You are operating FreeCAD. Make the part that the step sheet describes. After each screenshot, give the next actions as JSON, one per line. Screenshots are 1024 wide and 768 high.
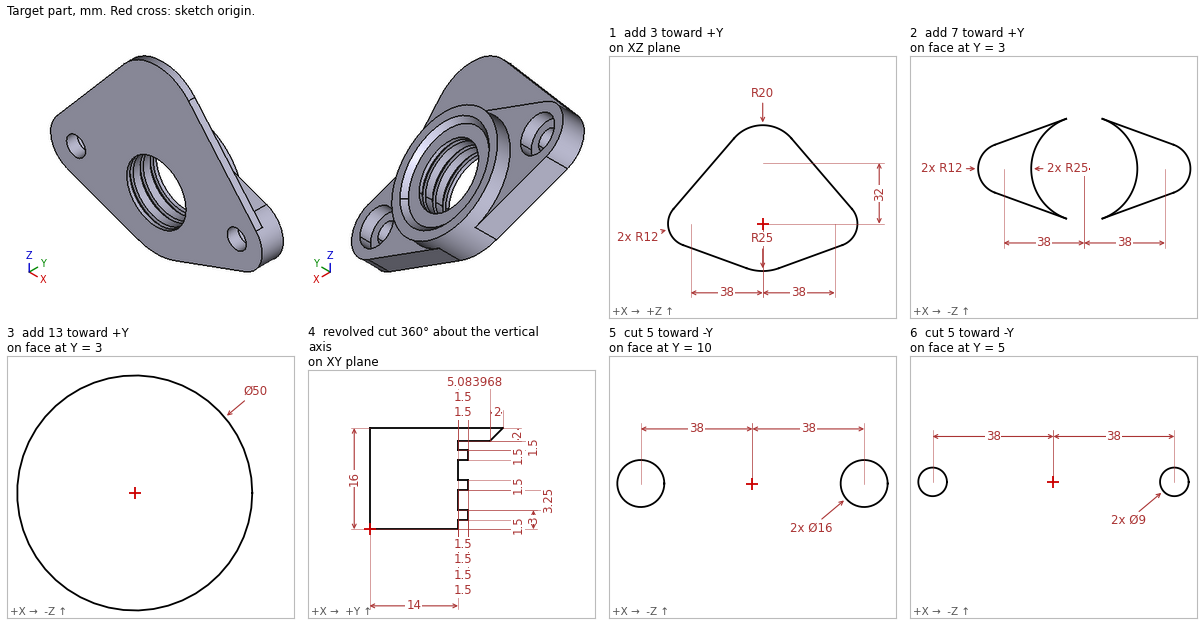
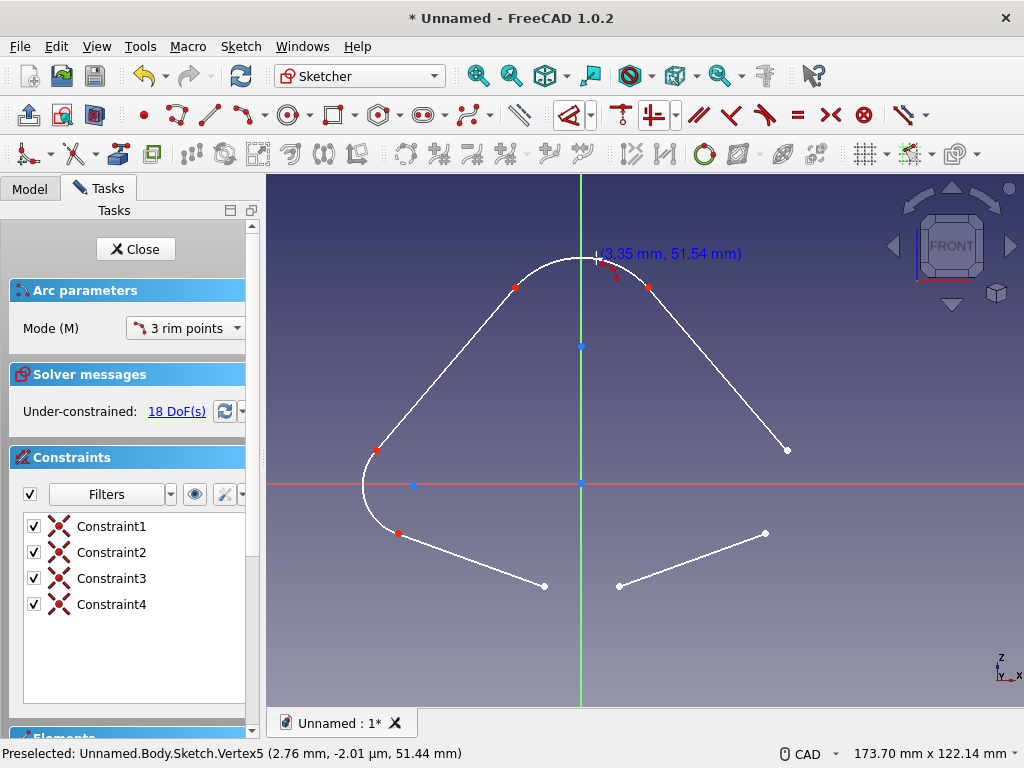
{"action": "left_click", "coordinate": [787, 451]}
{"action": "left_click", "coordinate": [765, 534]}
{"action": "left_click", "coordinate": [794, 507]}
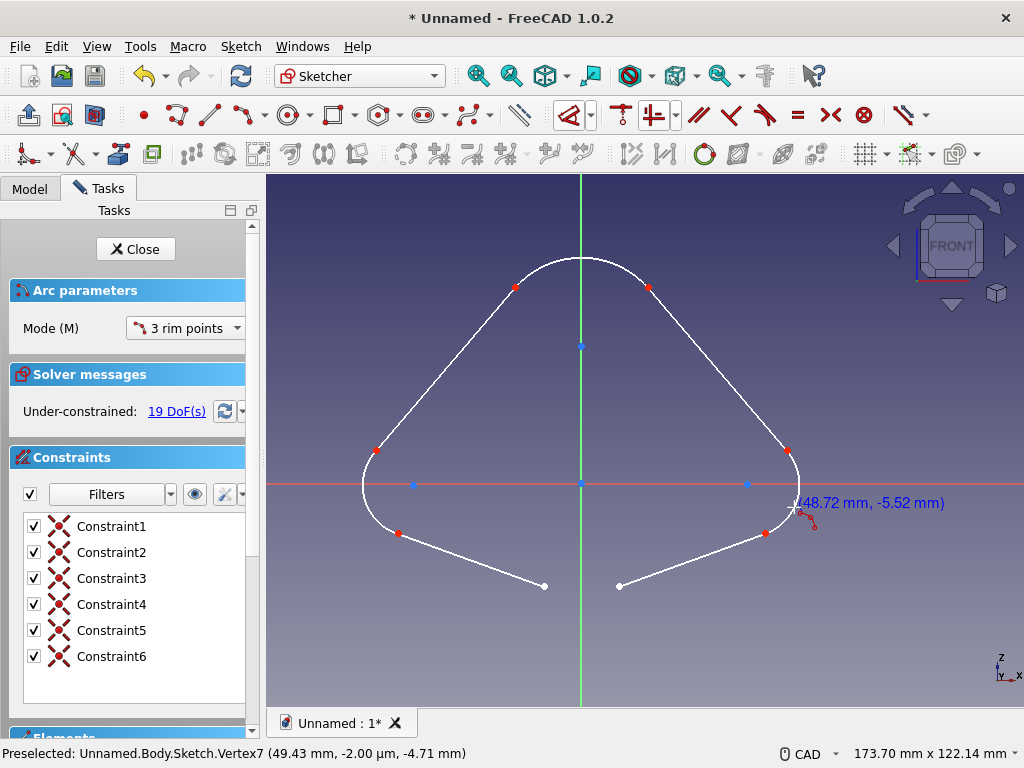
{"action": "left_click", "coordinate": [619, 587]}
{"action": "left_click", "coordinate": [544, 587]}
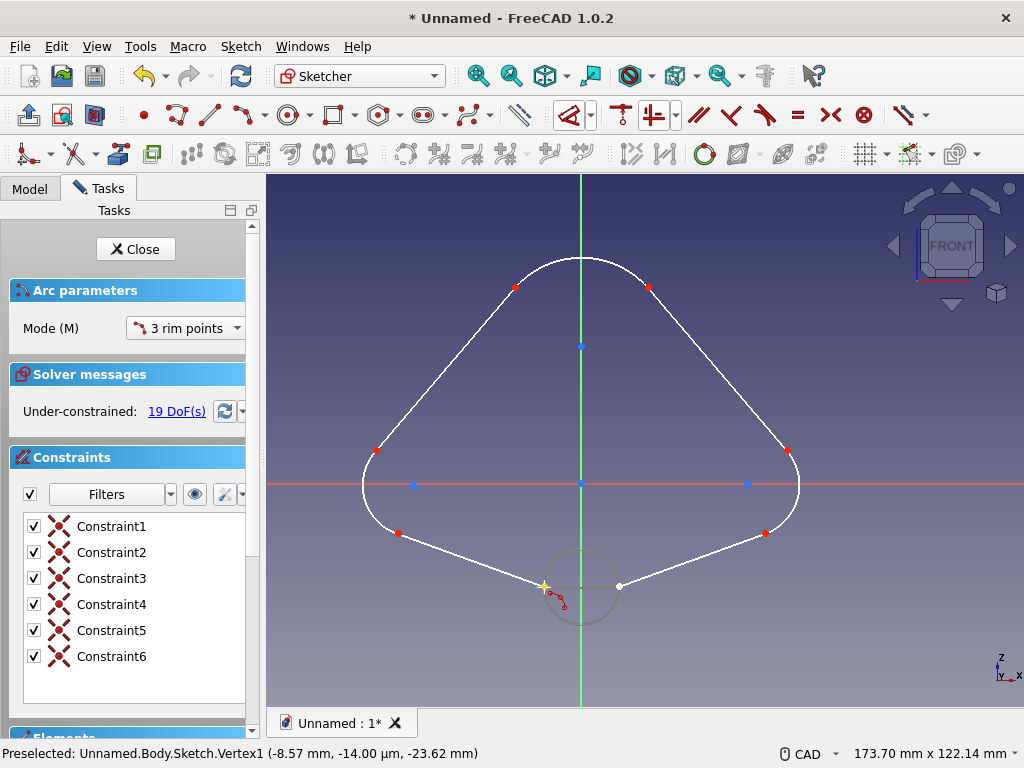
{"action": "scroll", "coordinate": [574, 593], "scroll_direction": "up", "scroll_amount": 5}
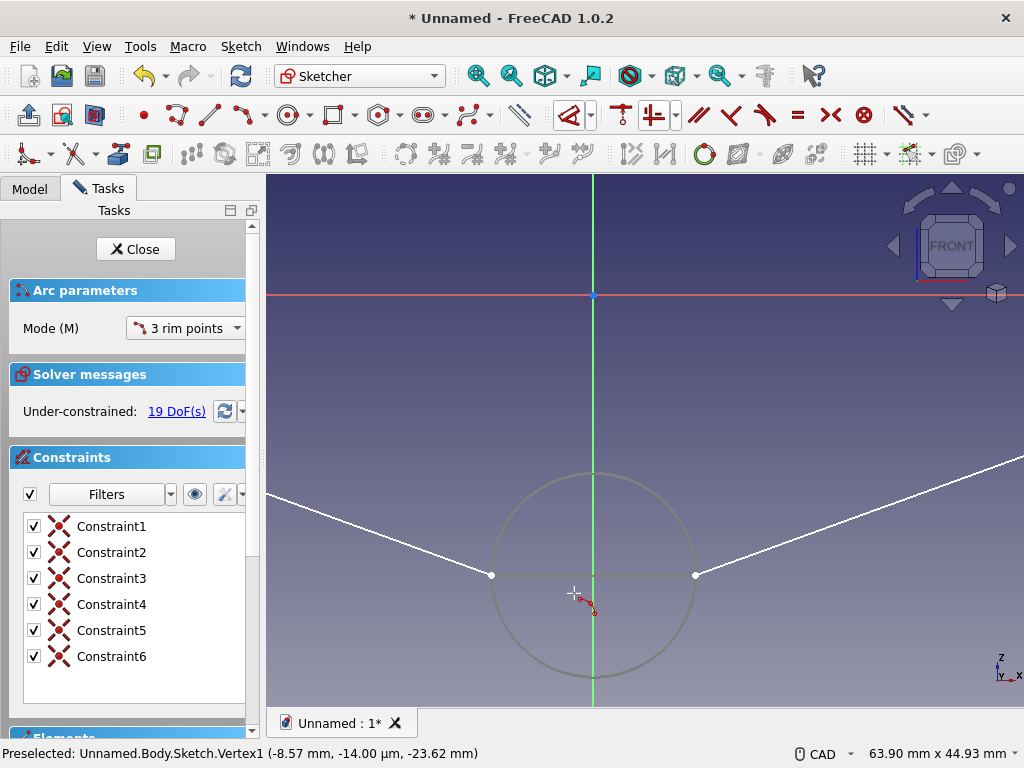
{"action": "left_click", "coordinate": [573, 591]}
{"action": "key", "text": "Escape"}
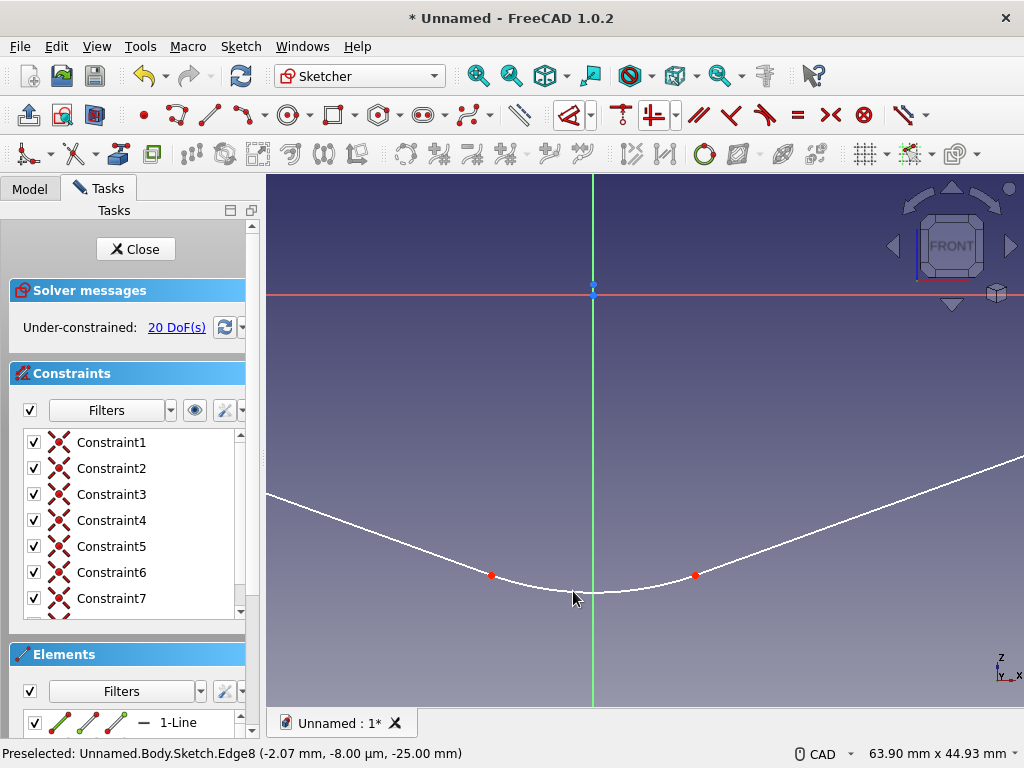
{"action": "left_click", "coordinate": [373, 532]}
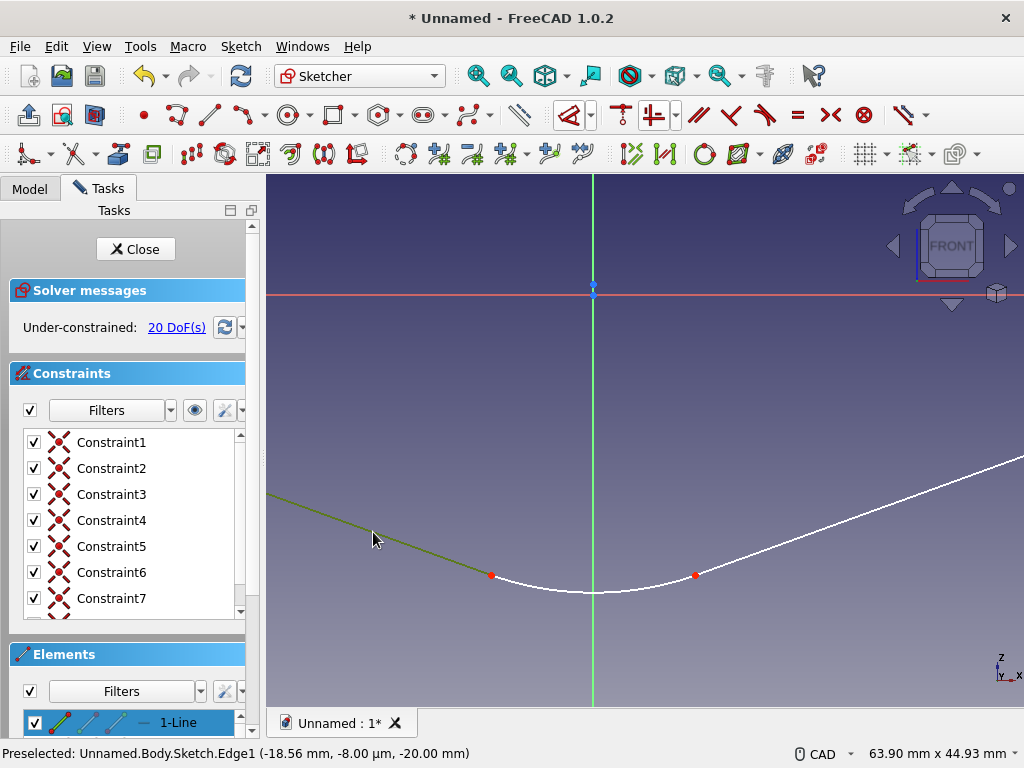
{"action": "scroll", "coordinate": [567, 618], "scroll_direction": "down", "scroll_amount": 5}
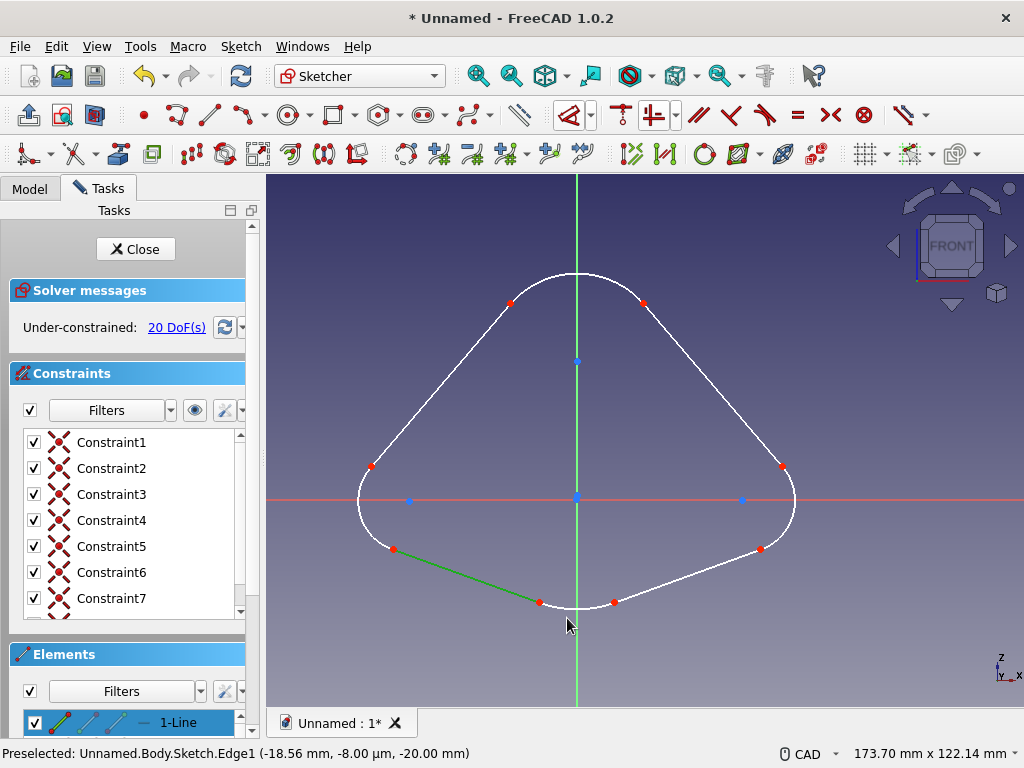
{"action": "scroll", "coordinate": [359, 494], "scroll_direction": "up", "scroll_amount": 5}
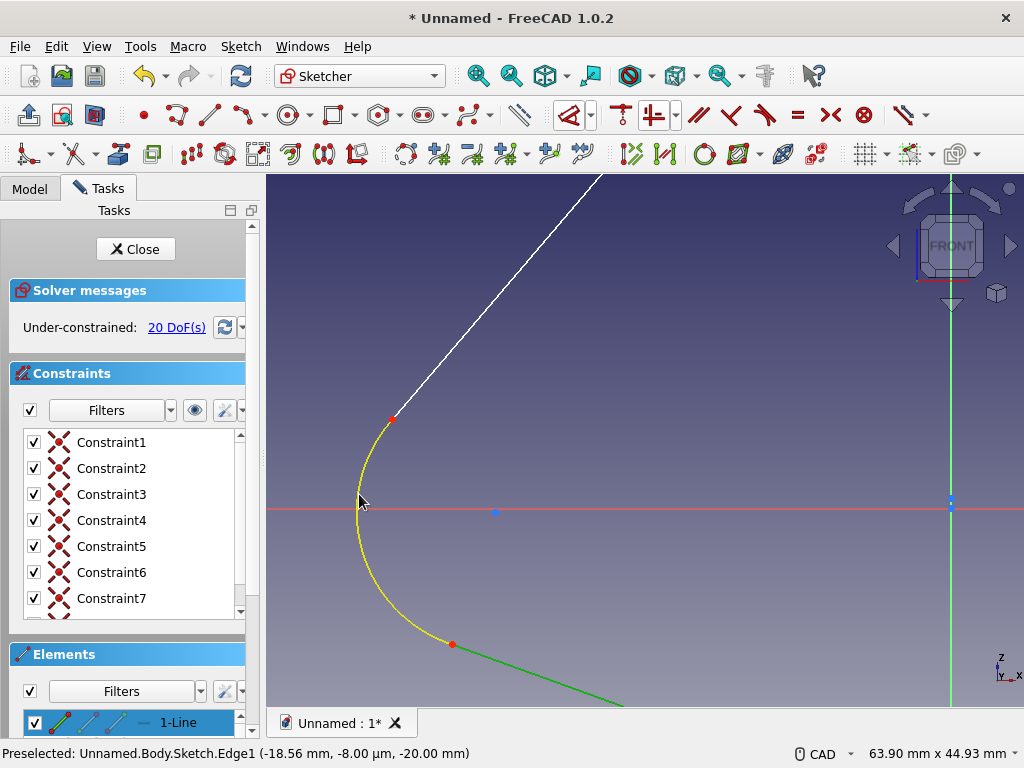
{"action": "left_click", "coordinate": [358, 493]}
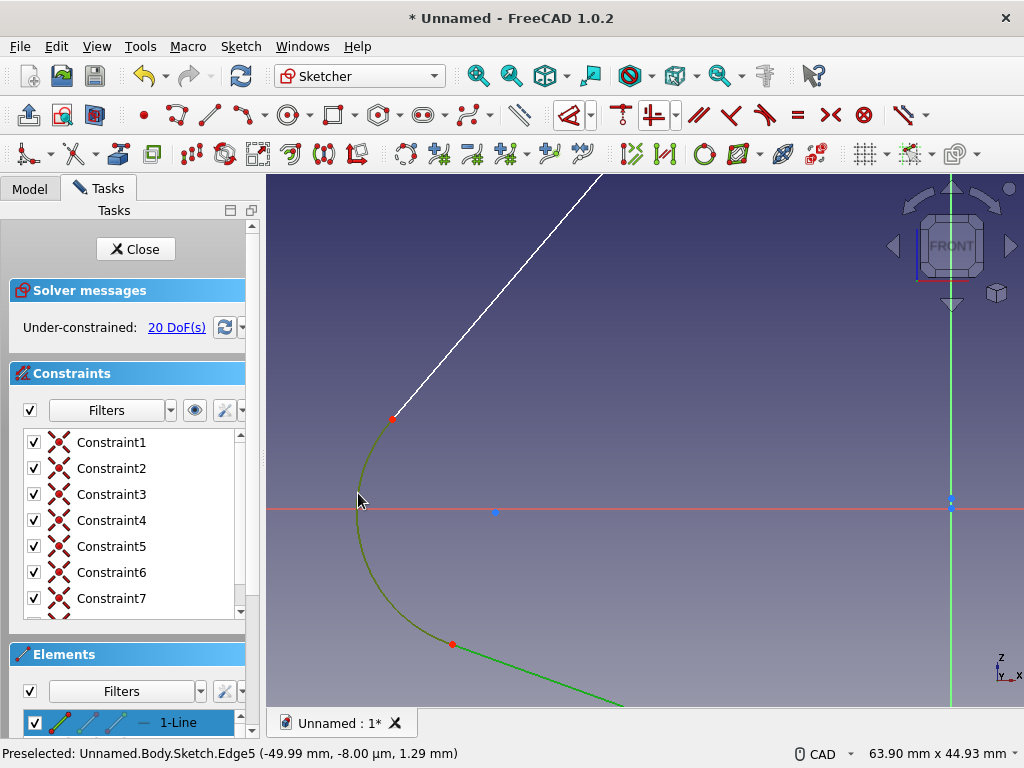
{"action": "left_click", "coordinate": [765, 116]}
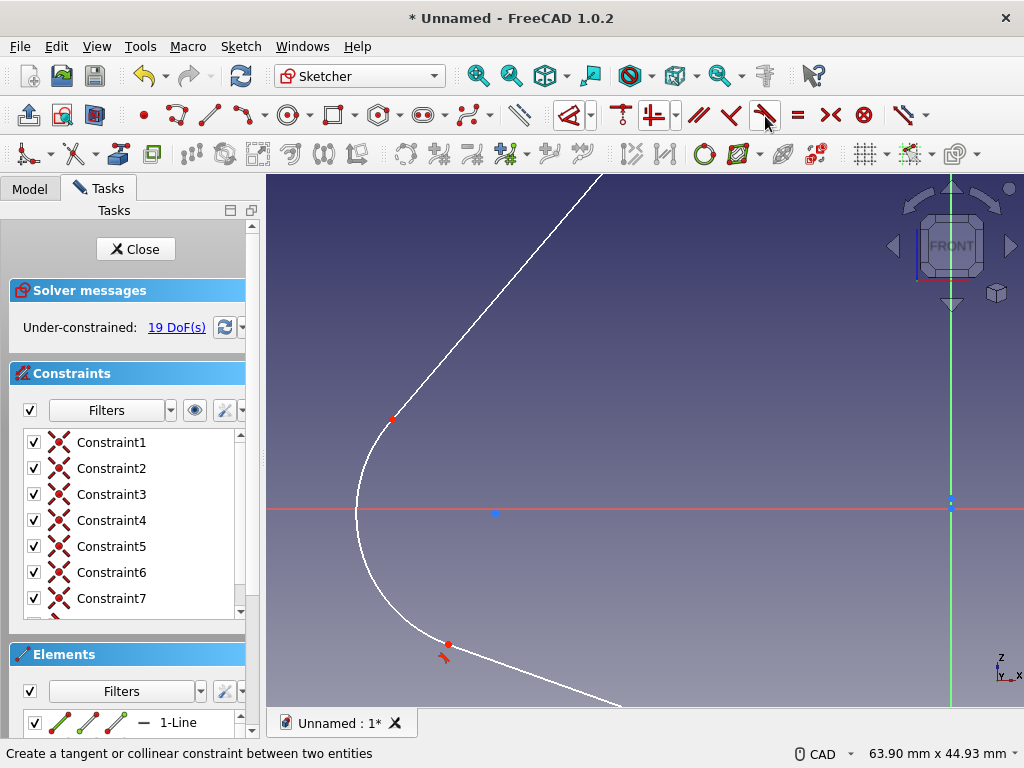
{"action": "left_click", "coordinate": [529, 674]}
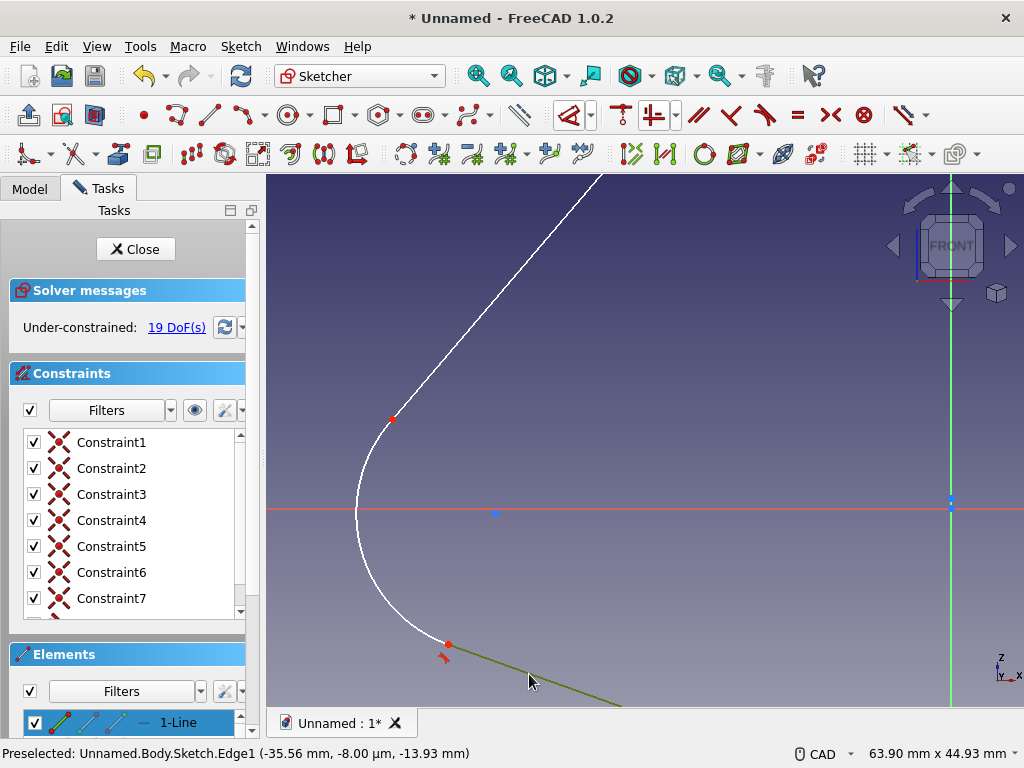
{"action": "scroll", "coordinate": [358, 494], "scroll_direction": "down", "scroll_amount": 5}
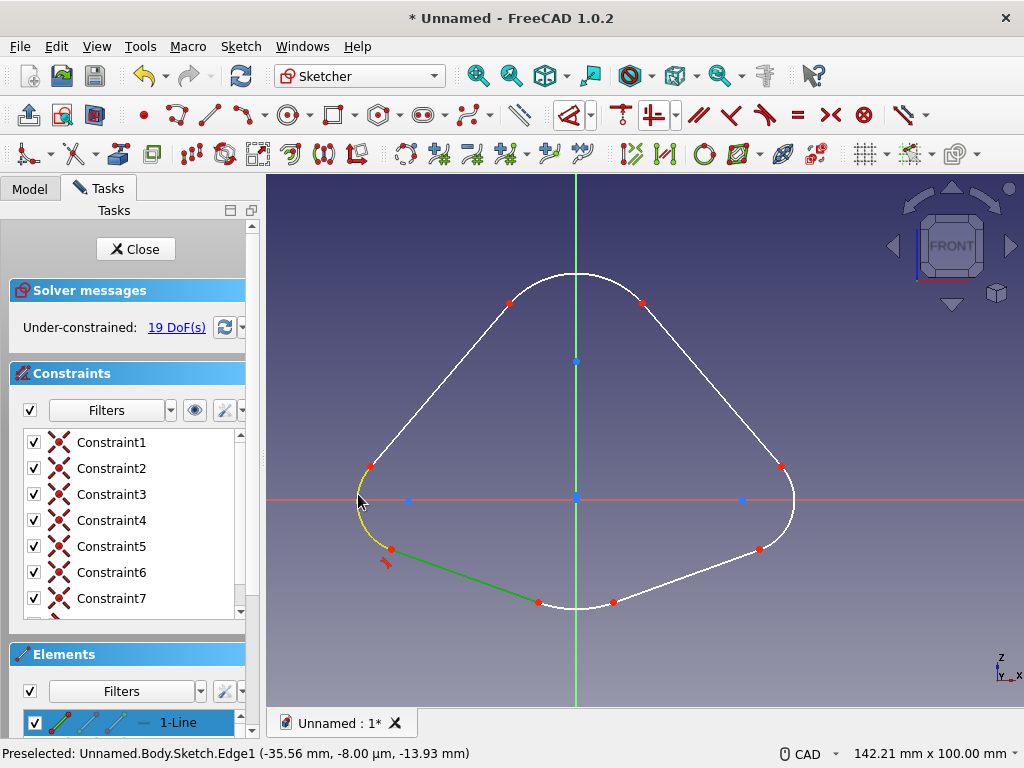
{"action": "left_click", "coordinate": [561, 608]}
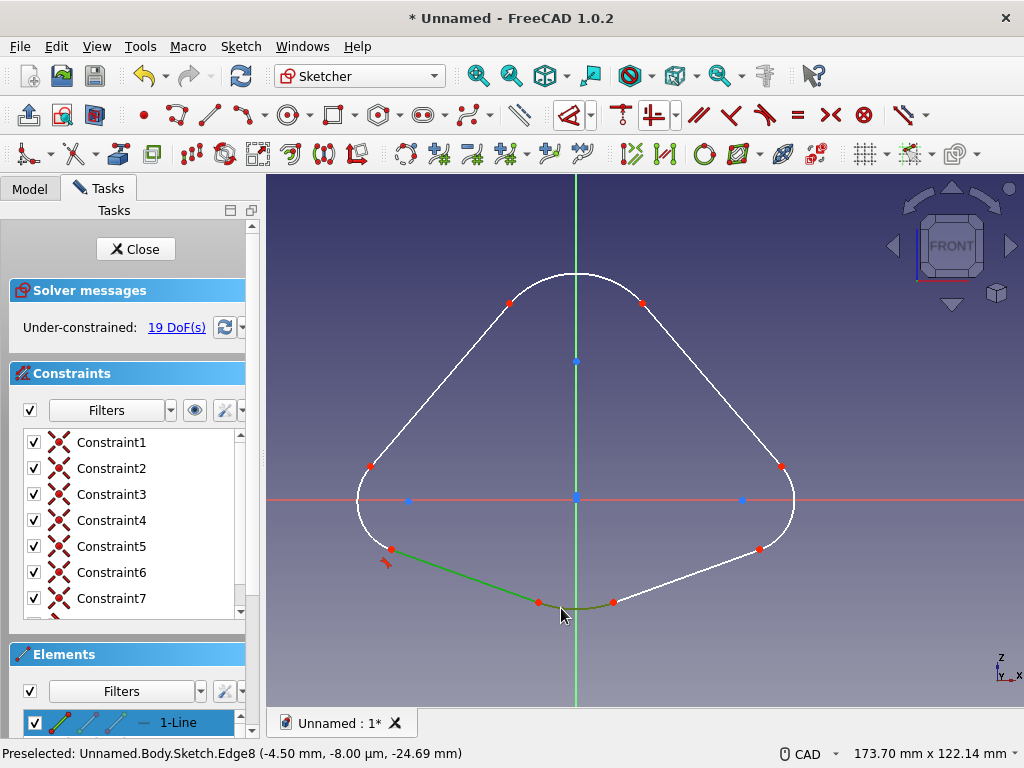
{"action": "left_click", "coordinate": [765, 116]}